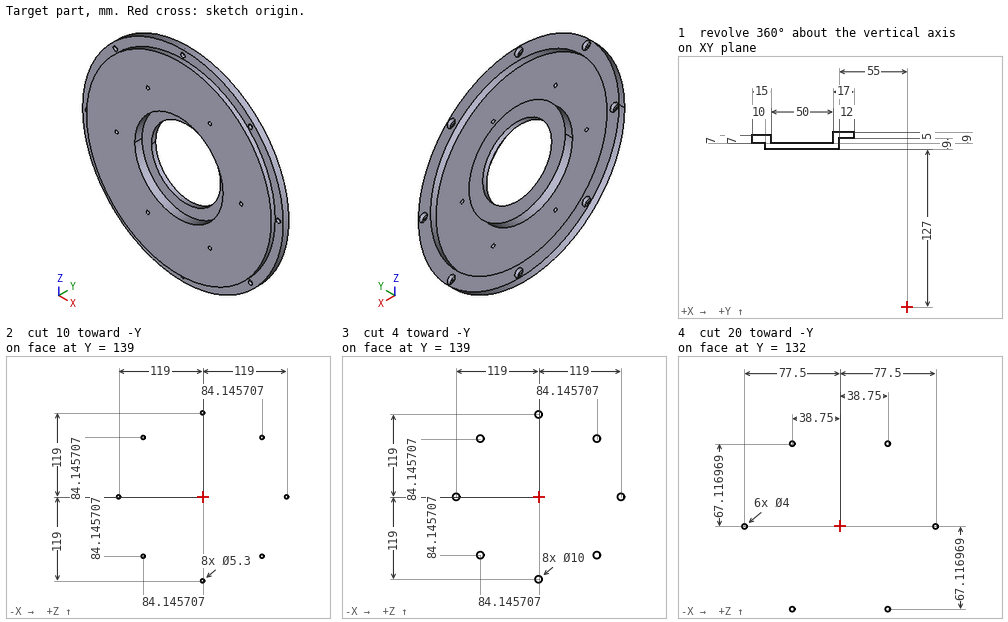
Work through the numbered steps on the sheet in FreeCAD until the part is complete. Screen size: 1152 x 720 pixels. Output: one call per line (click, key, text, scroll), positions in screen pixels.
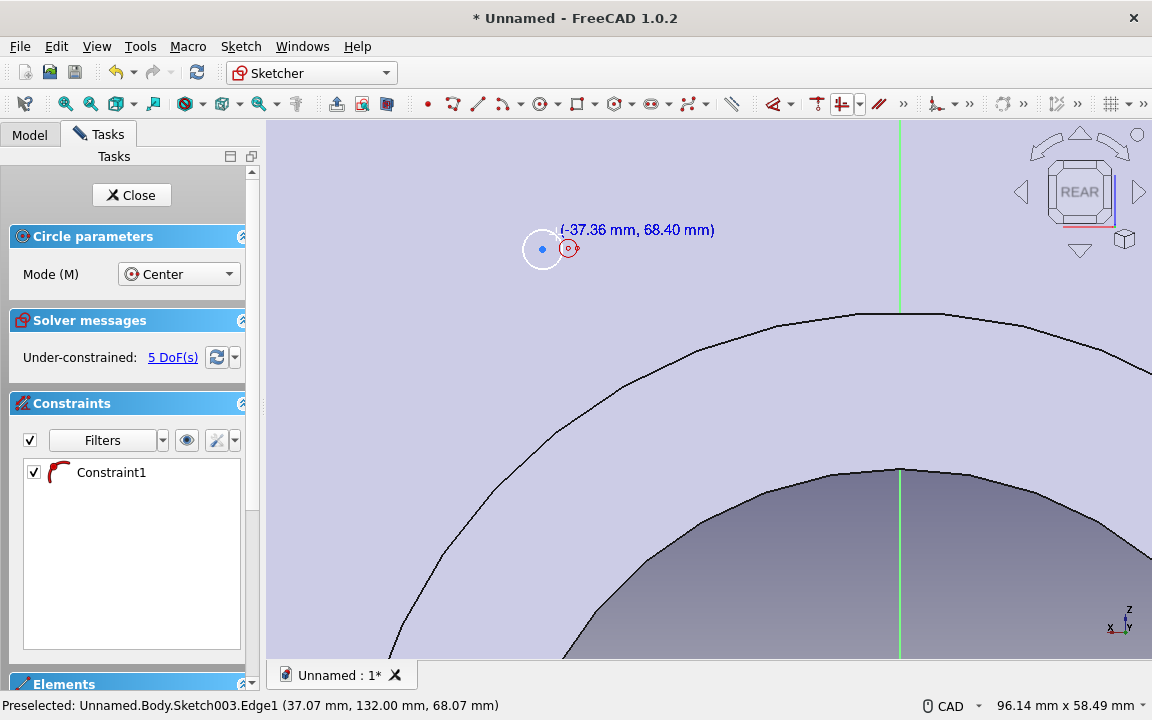
scroll(555, 234, down, 7)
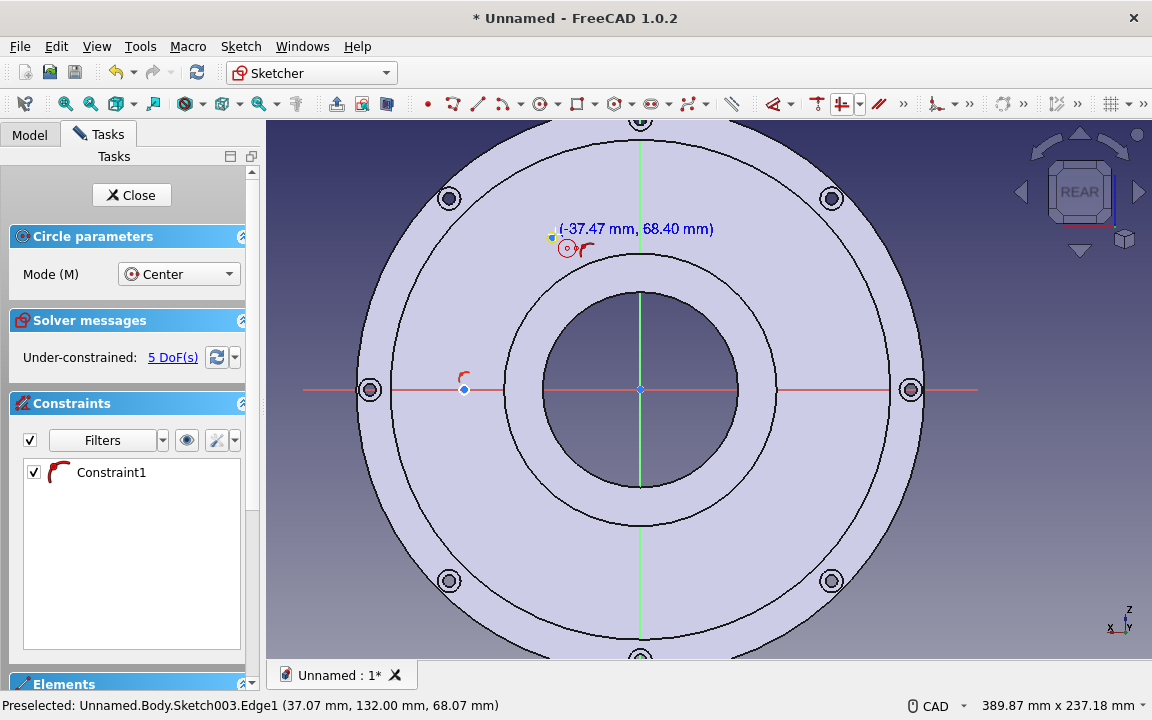
scroll(728, 237, up, 9)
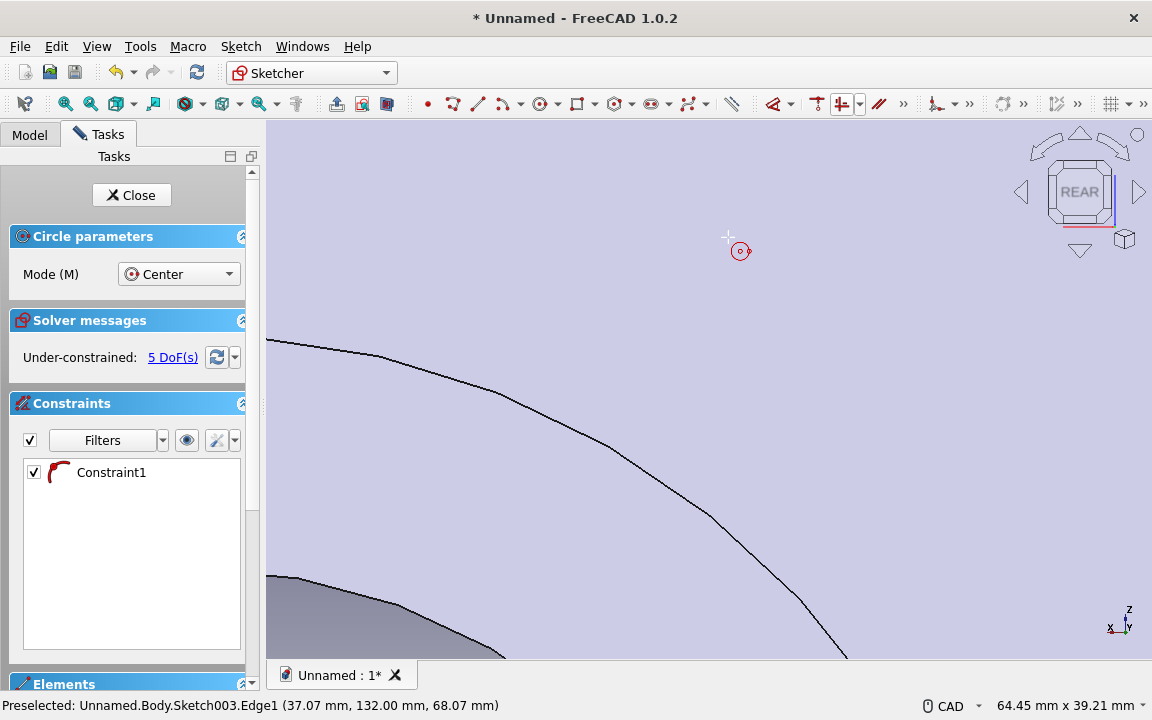
scroll(729, 237, down, 9)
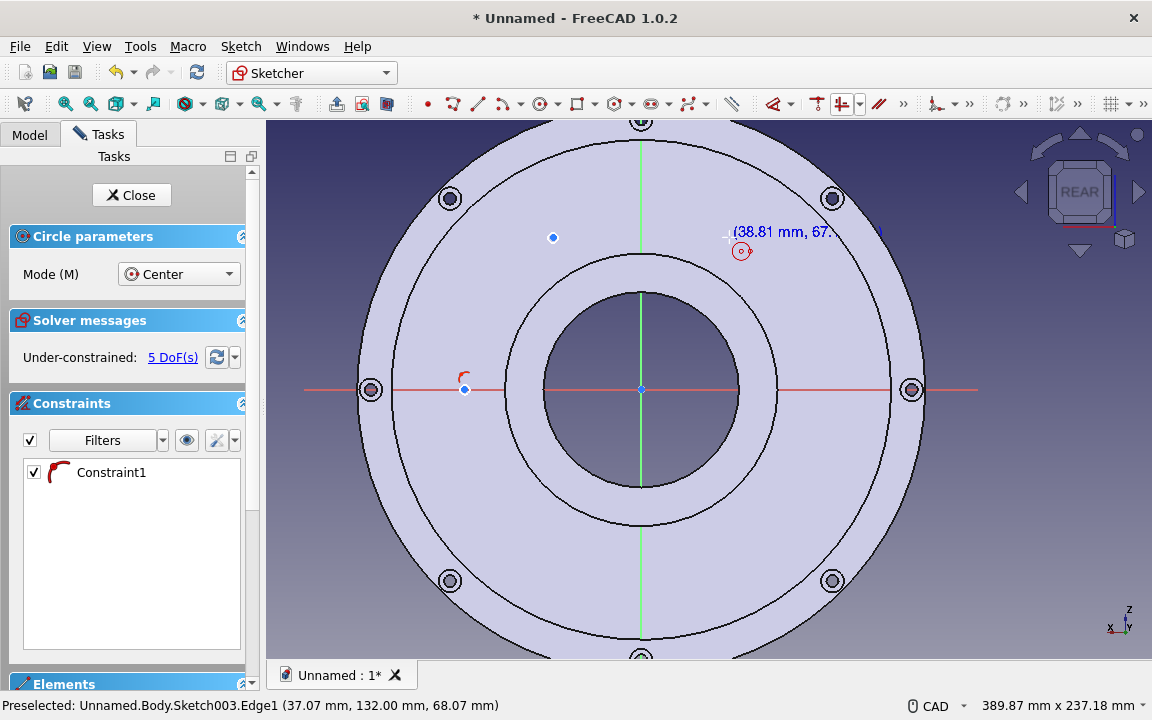
click(729, 237)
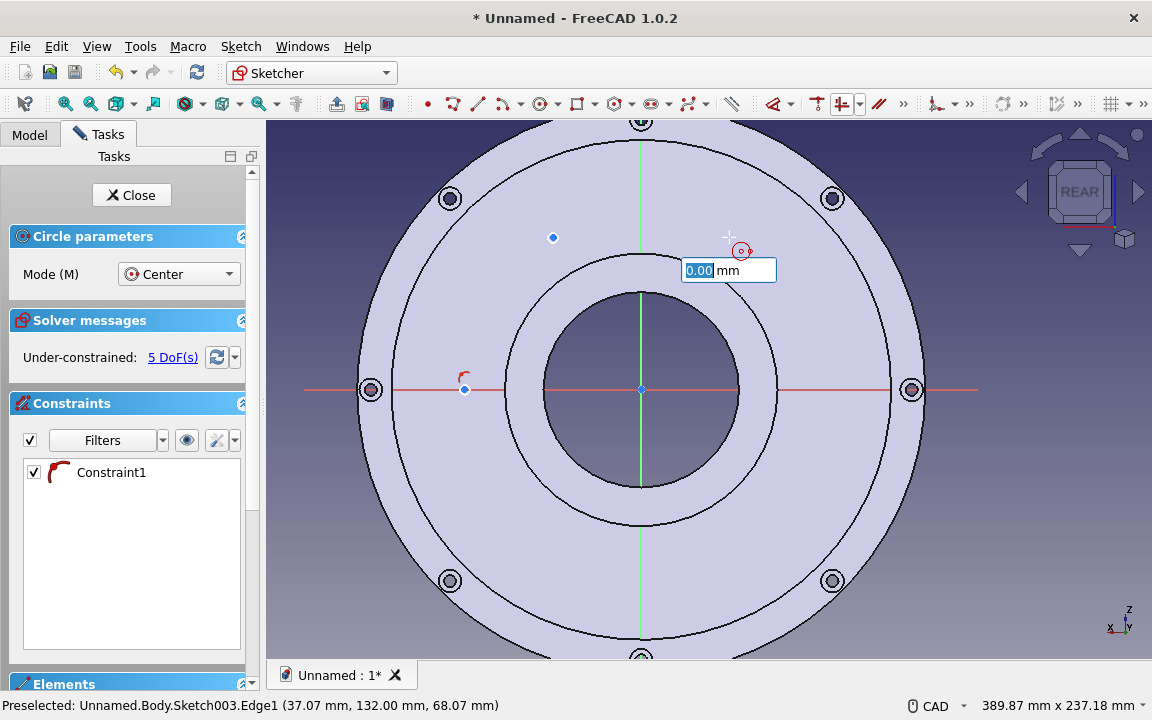
scroll(733, 234, up, 7)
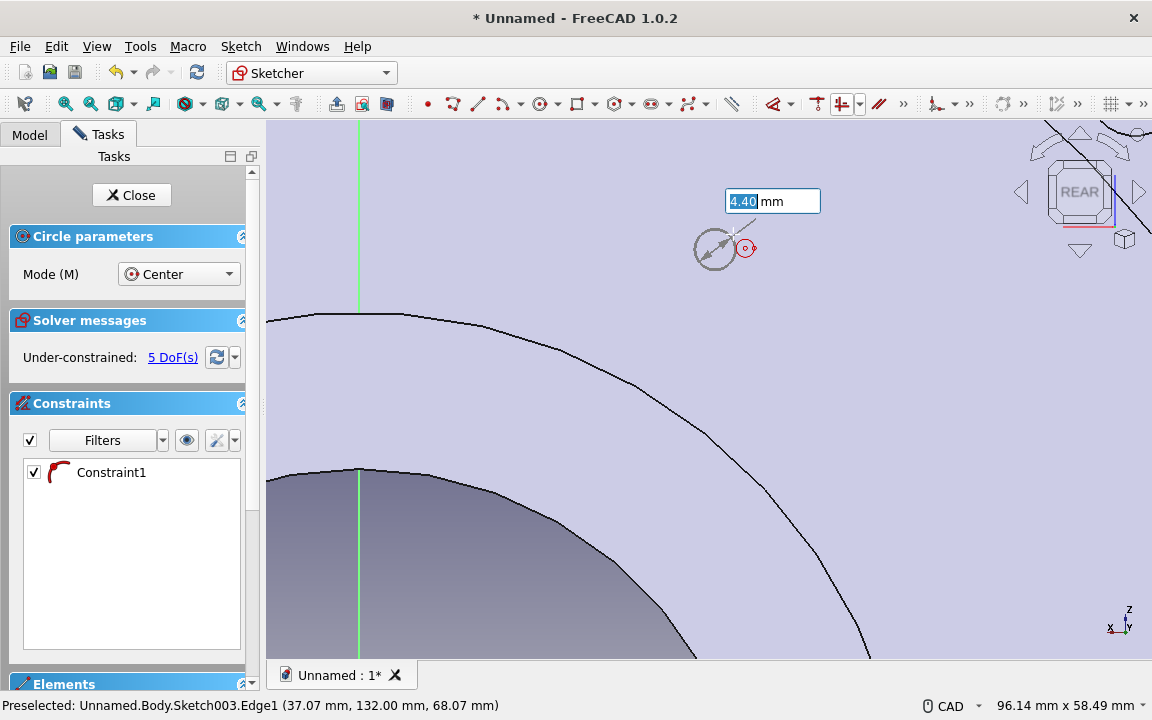
click(729, 234)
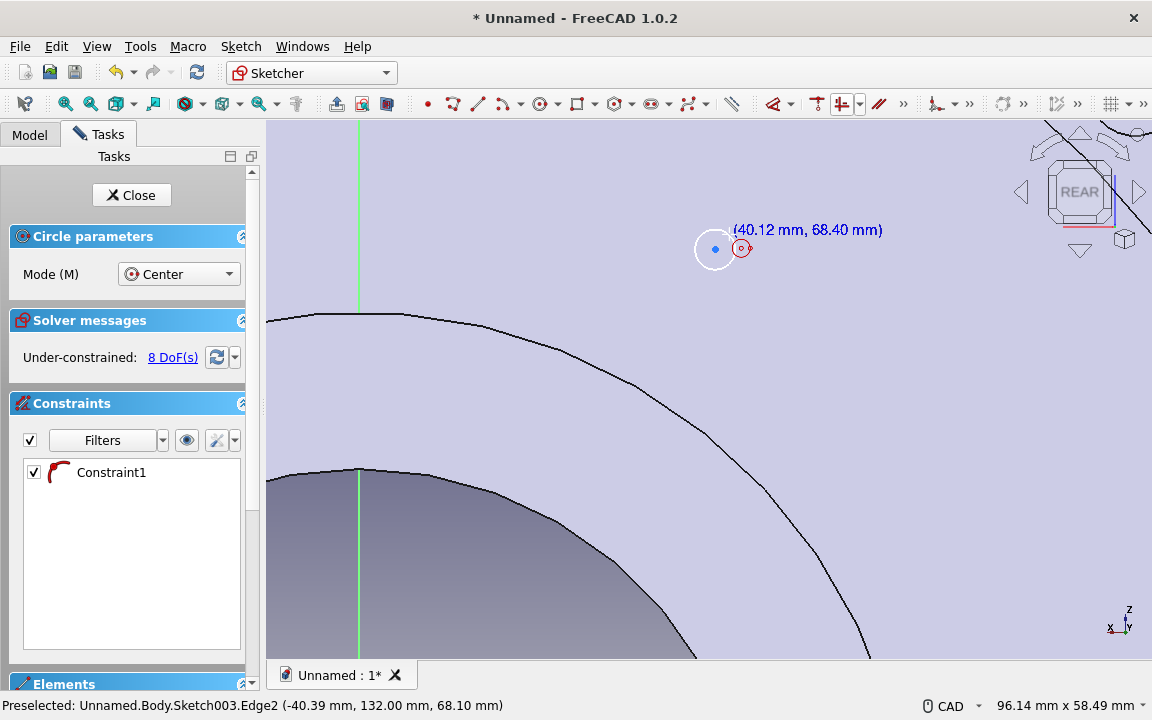
scroll(733, 234, down, 7)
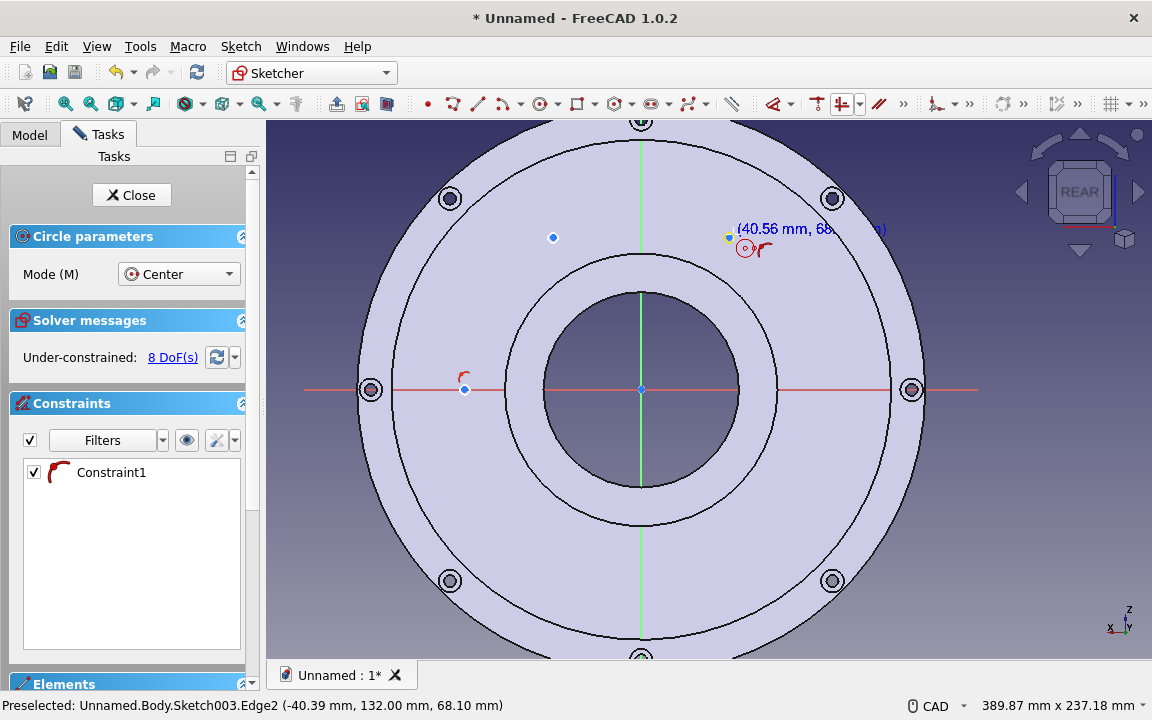
scroll(817, 390, up, 9)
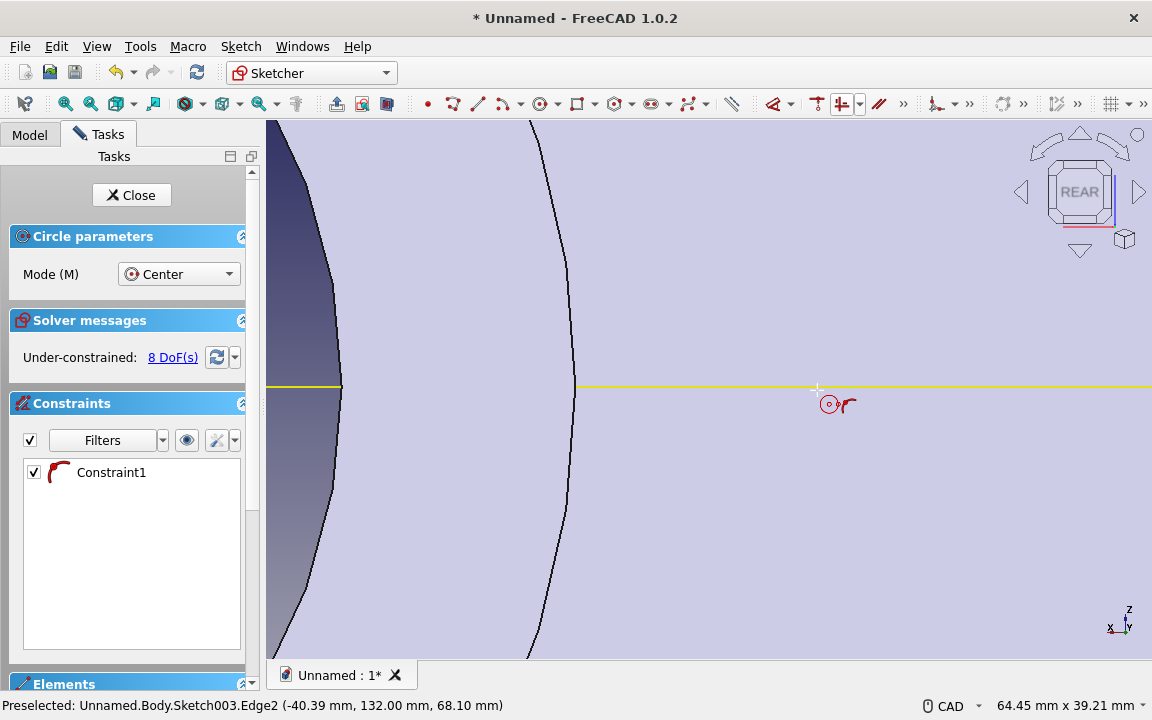
scroll(817, 390, down, 9)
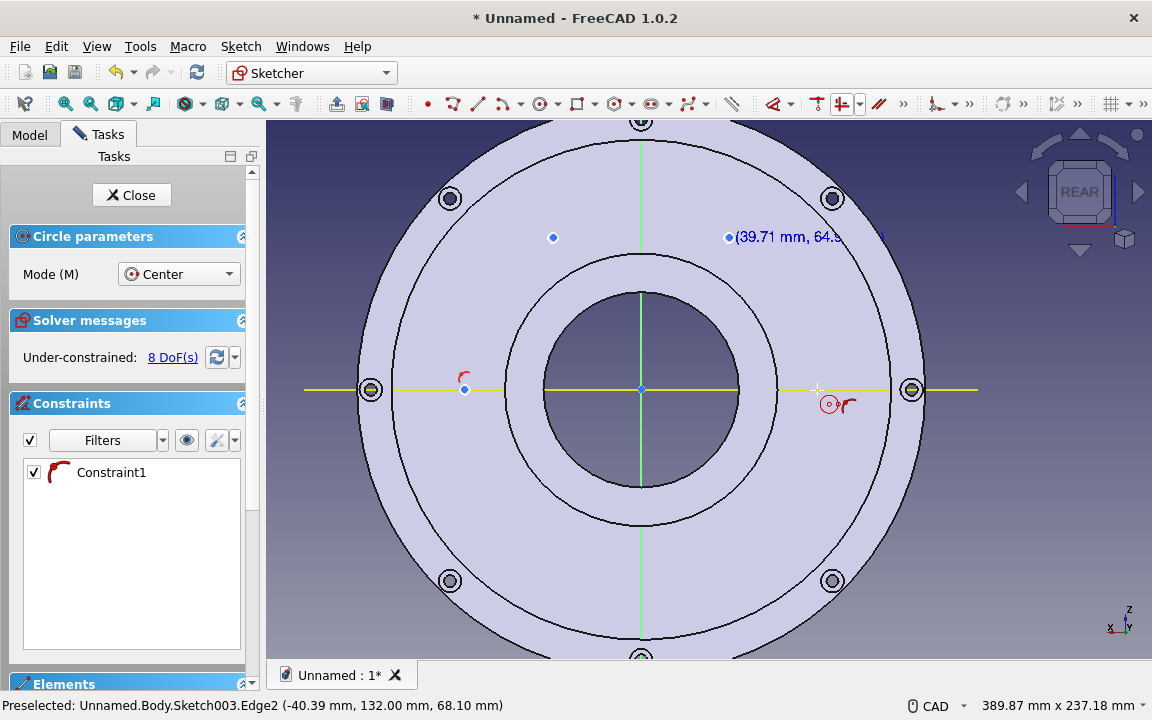
click(817, 390)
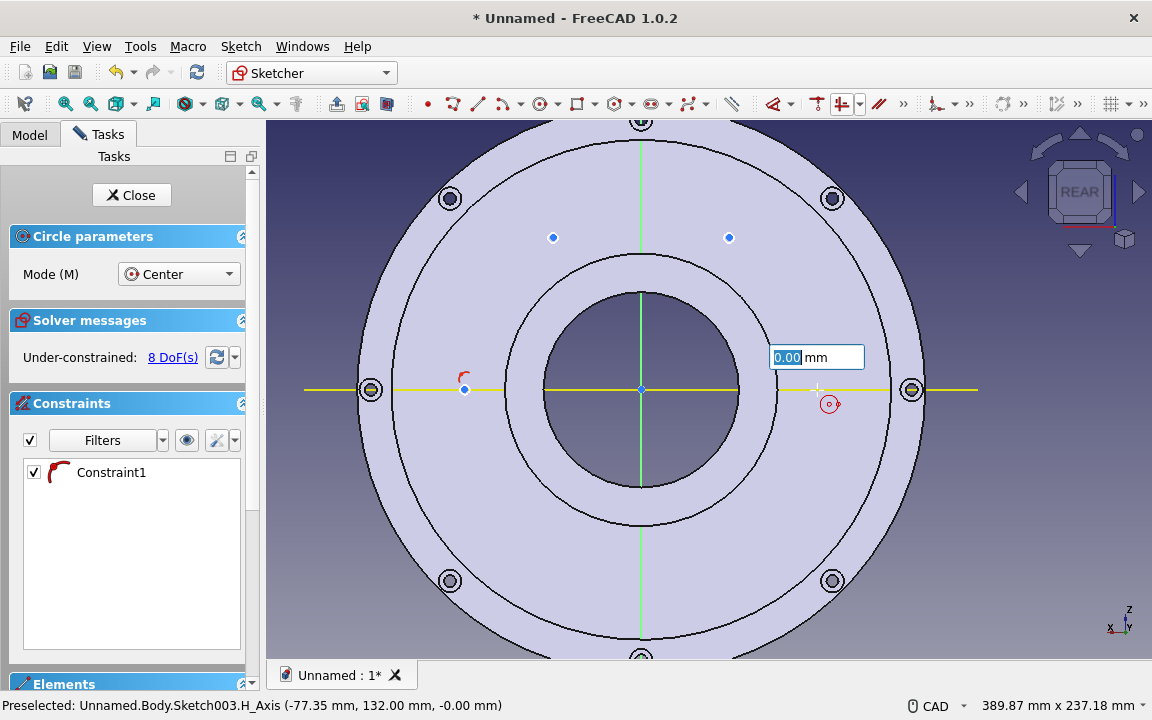
scroll(819, 386, up, 7)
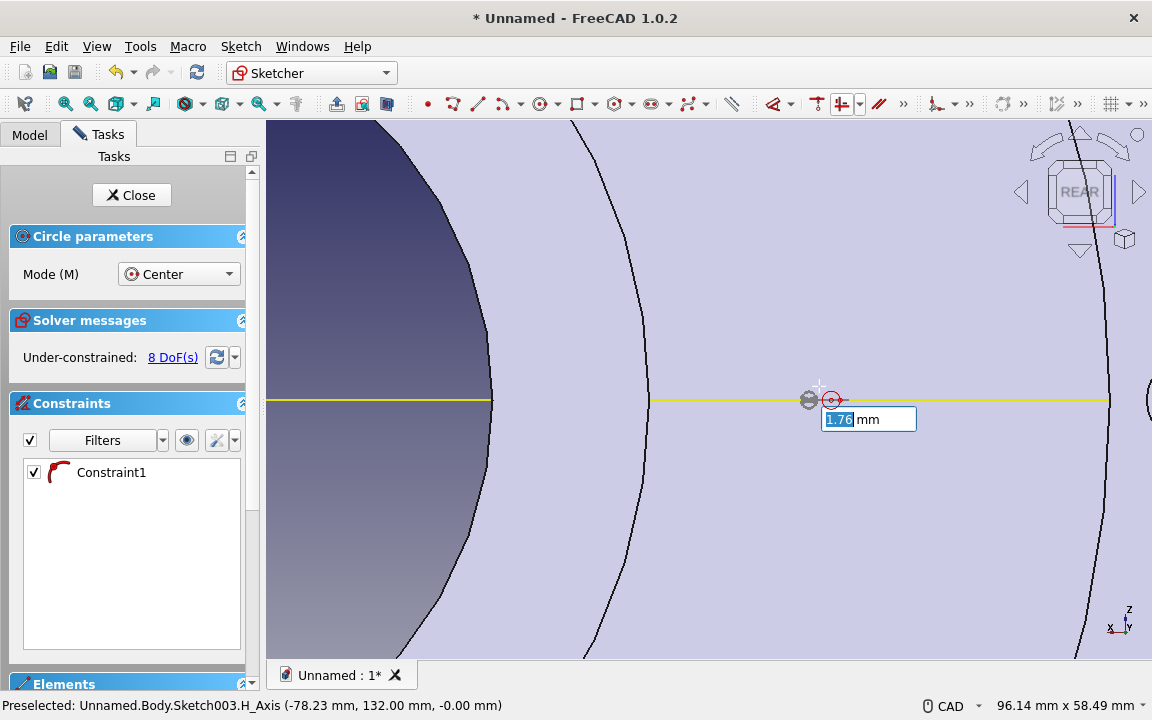
click(817, 383)